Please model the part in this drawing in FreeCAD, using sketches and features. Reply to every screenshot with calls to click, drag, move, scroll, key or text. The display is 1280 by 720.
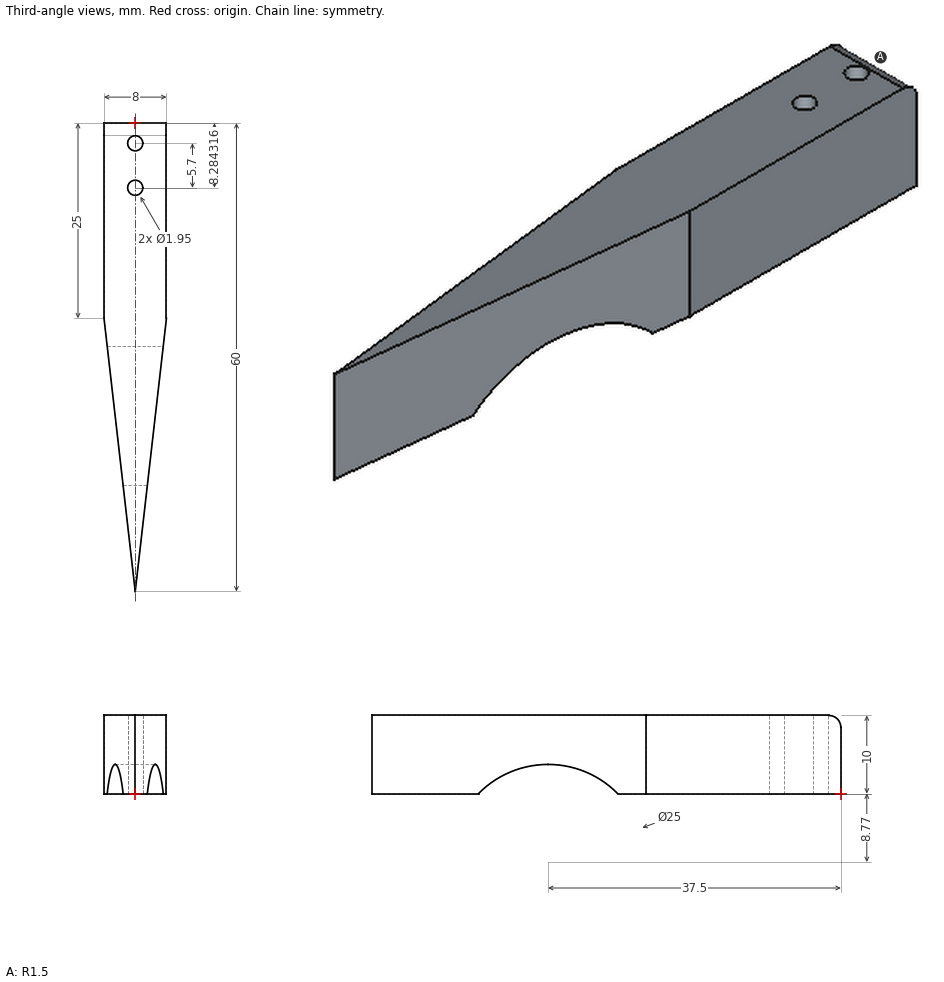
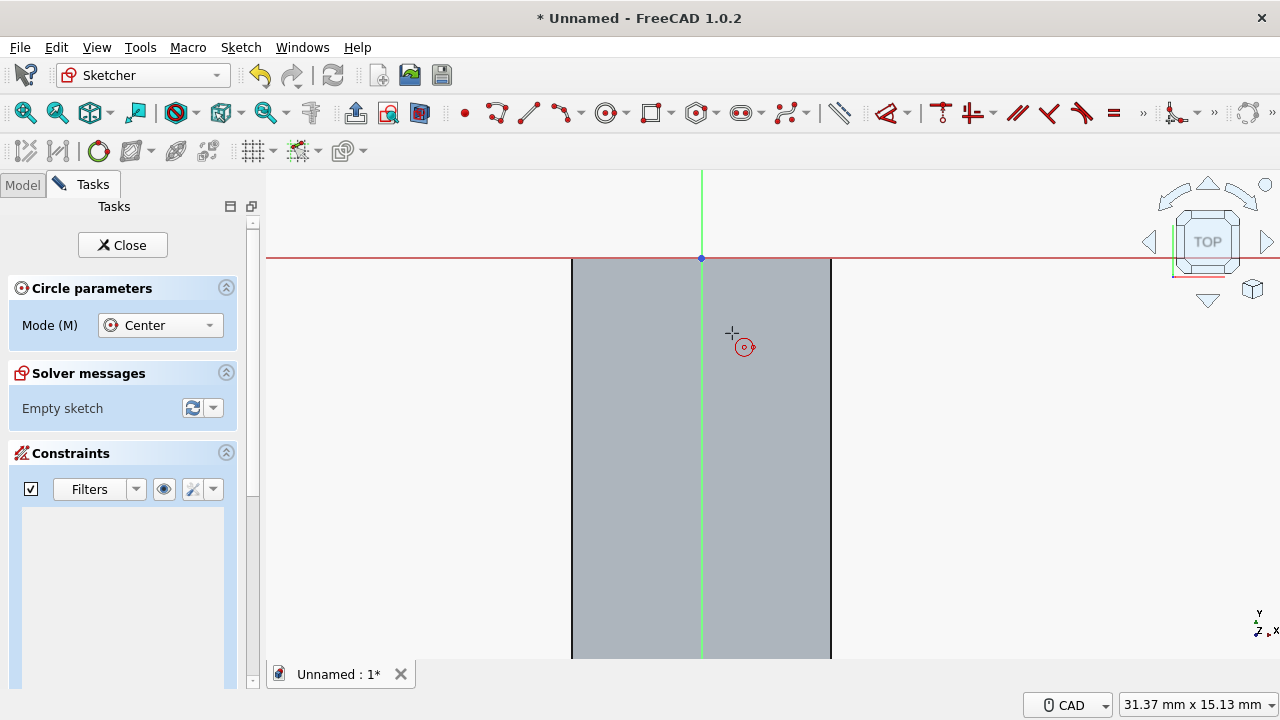
click(702, 526)
move(724, 504)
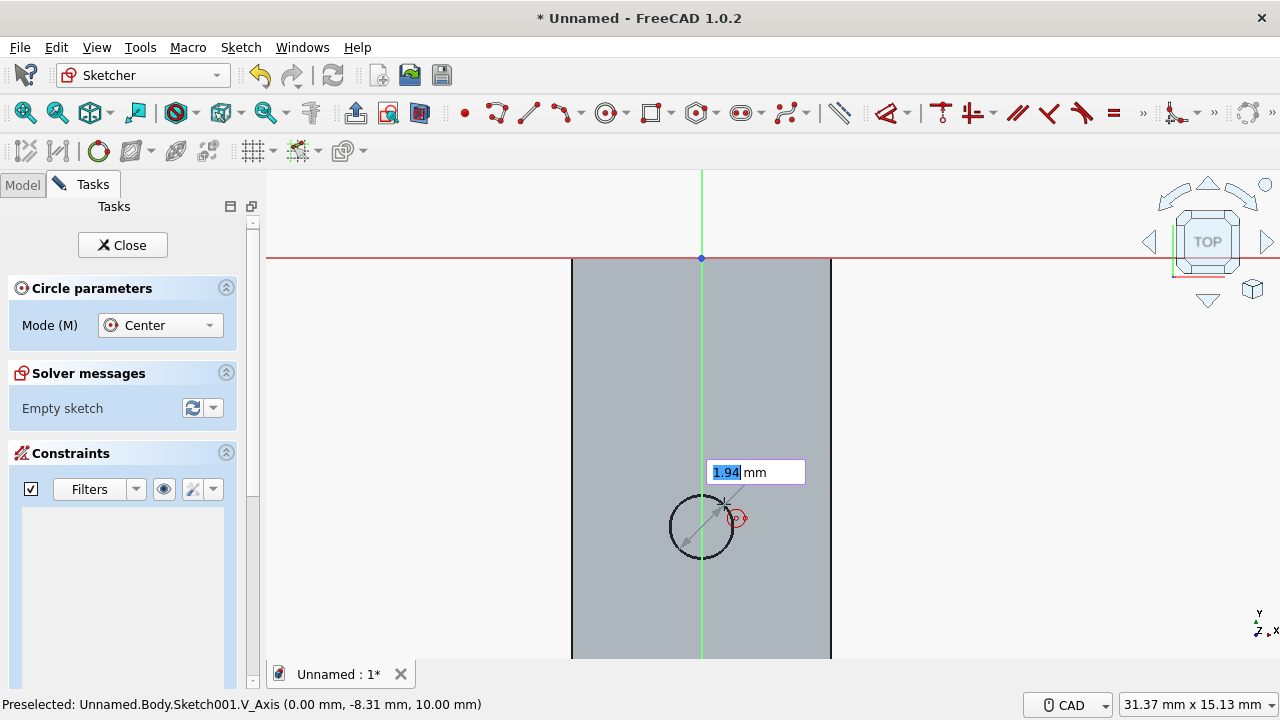
text(1.95)
key(Return)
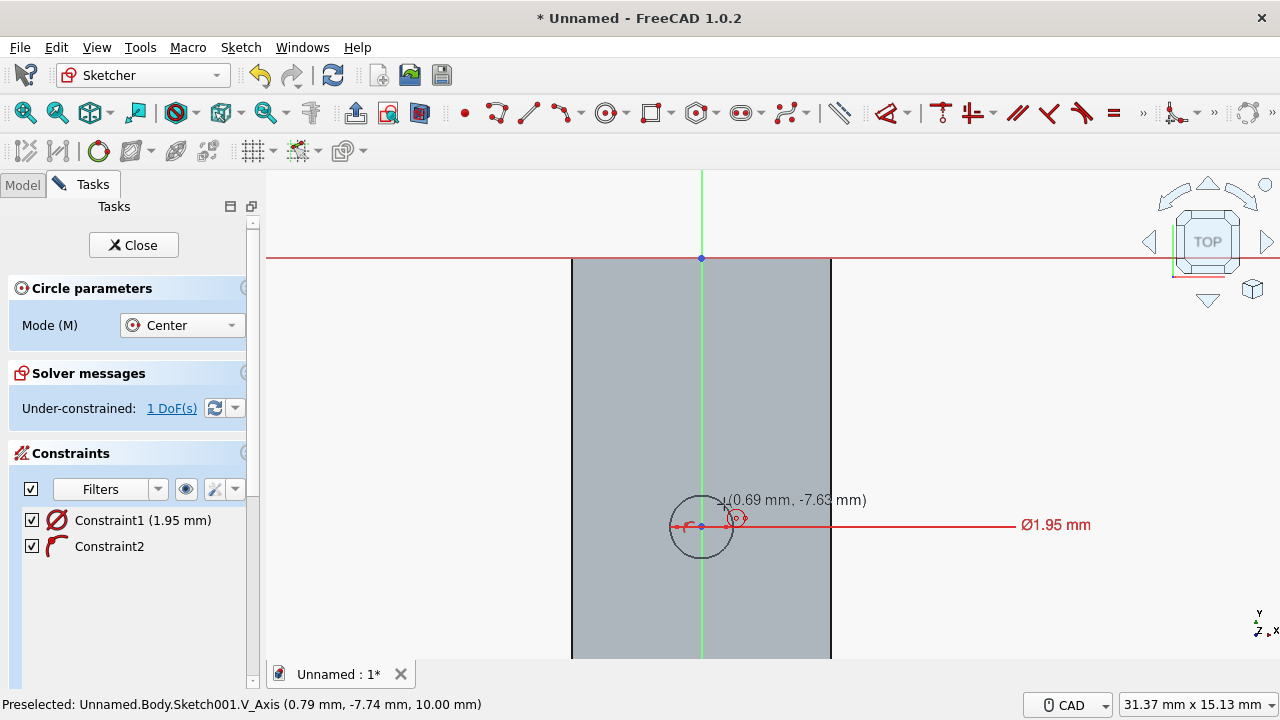
click(702, 342)
move(724, 320)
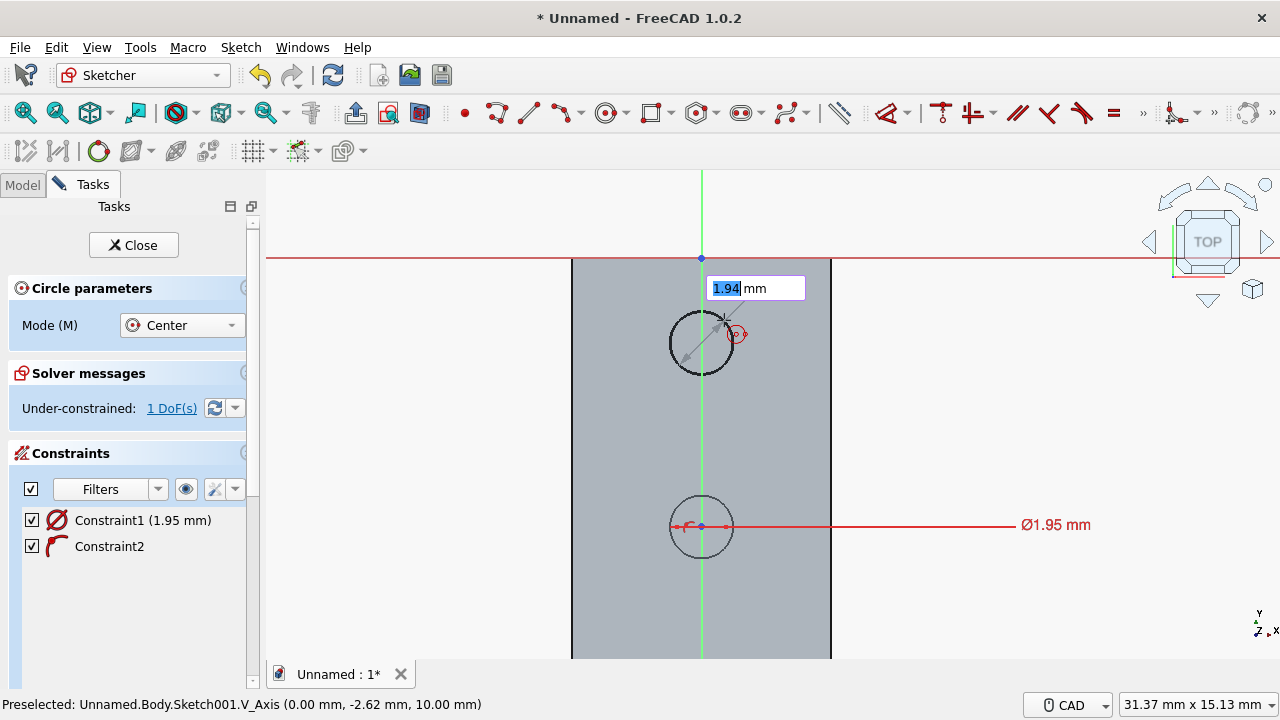
text(1.95)
key(Return)
key(Escape)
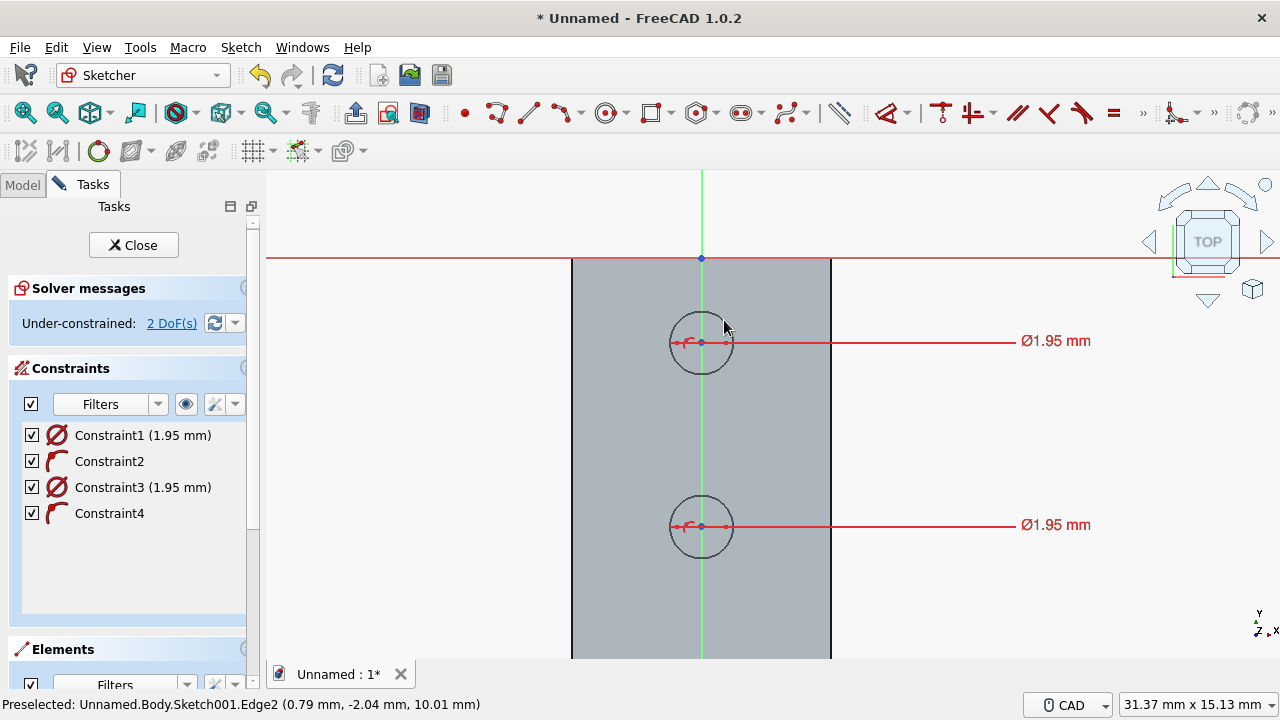
click(886, 114)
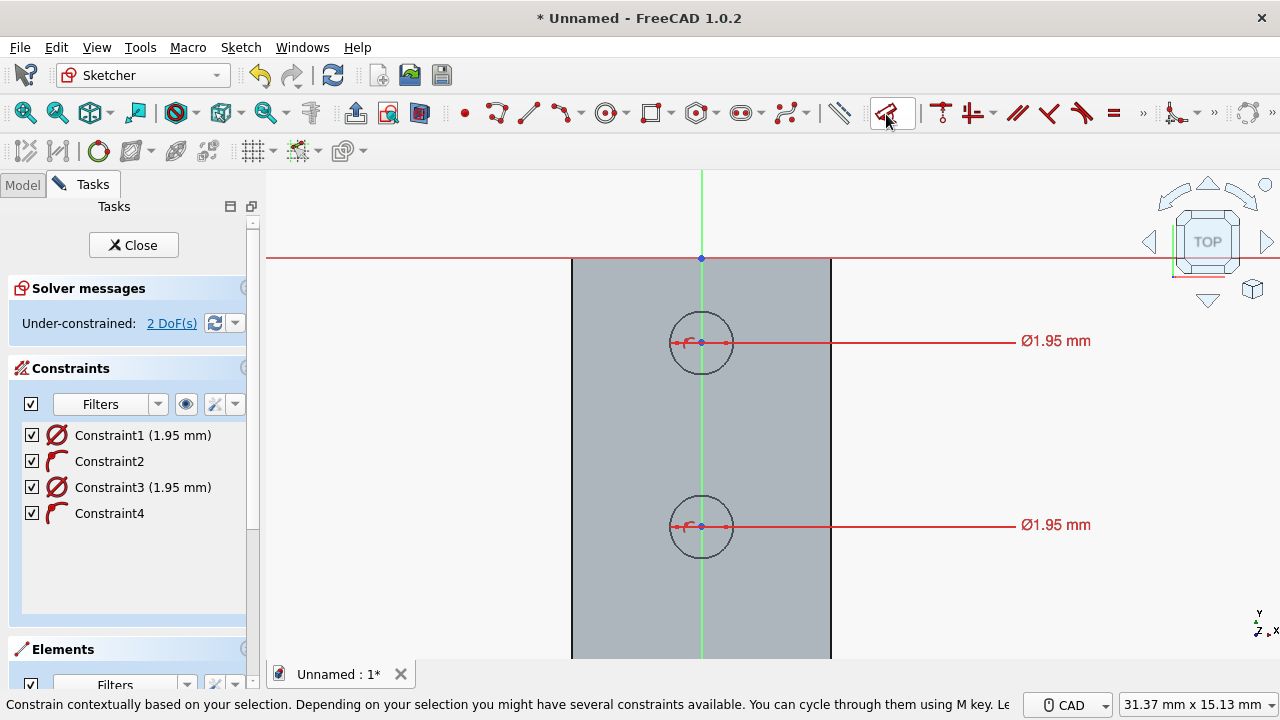
click(702, 527)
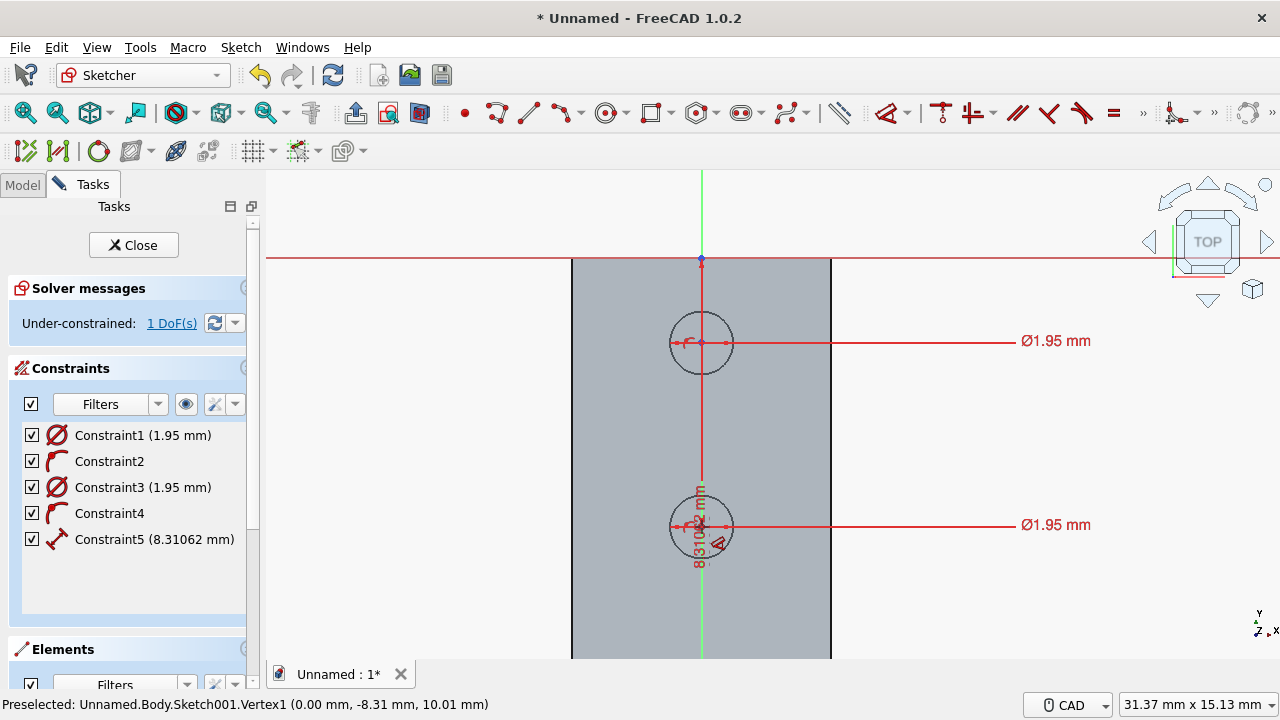
click(702, 343)
click(736, 435)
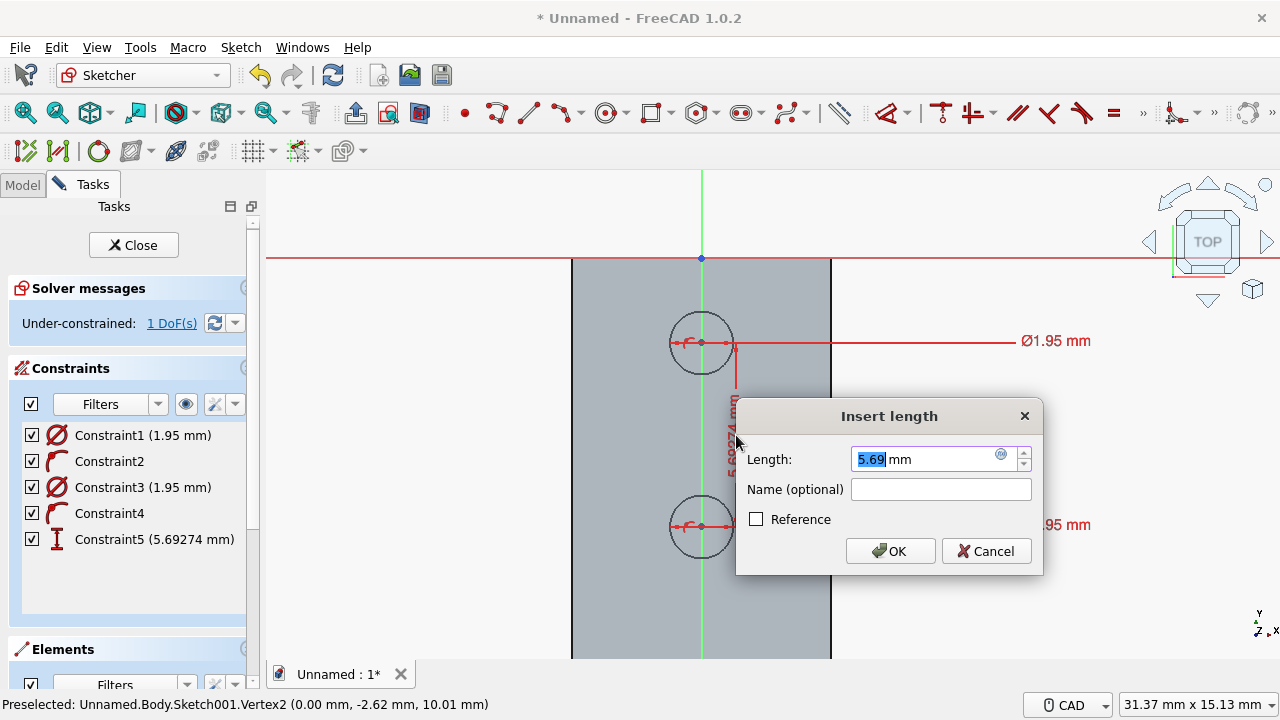
text(5.7)
key(Return)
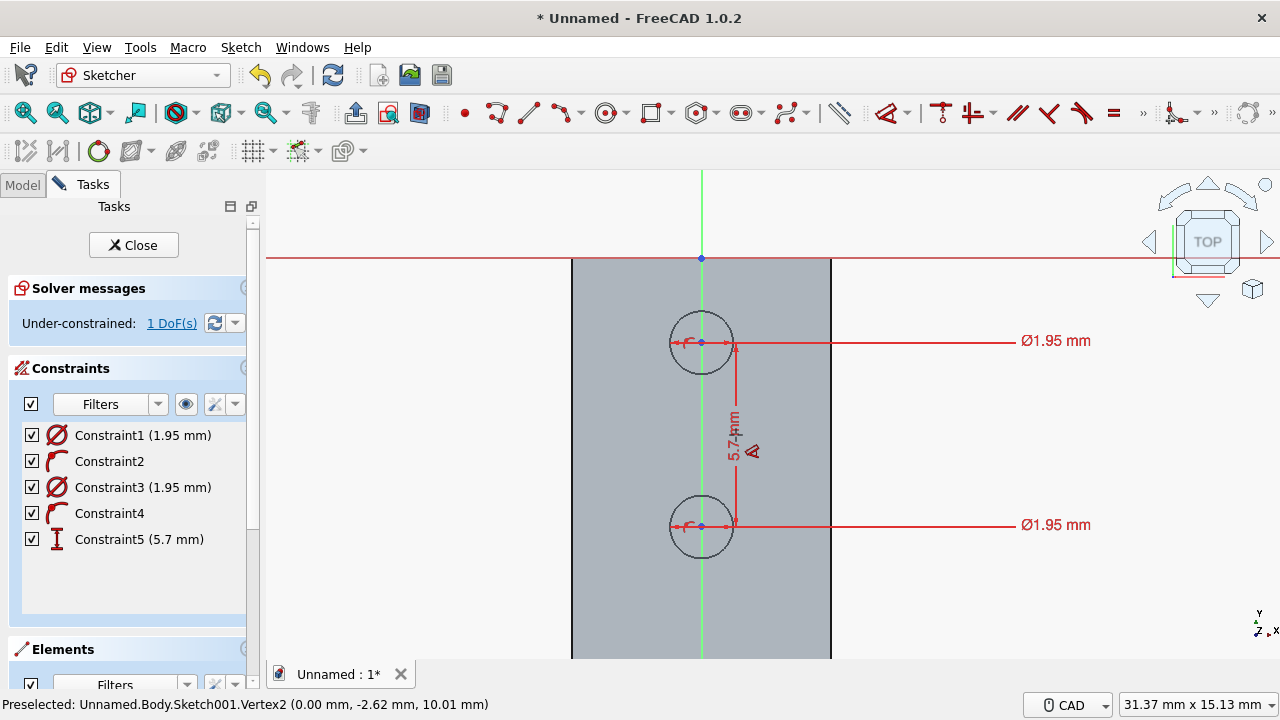
click(702, 527)
click(736, 393)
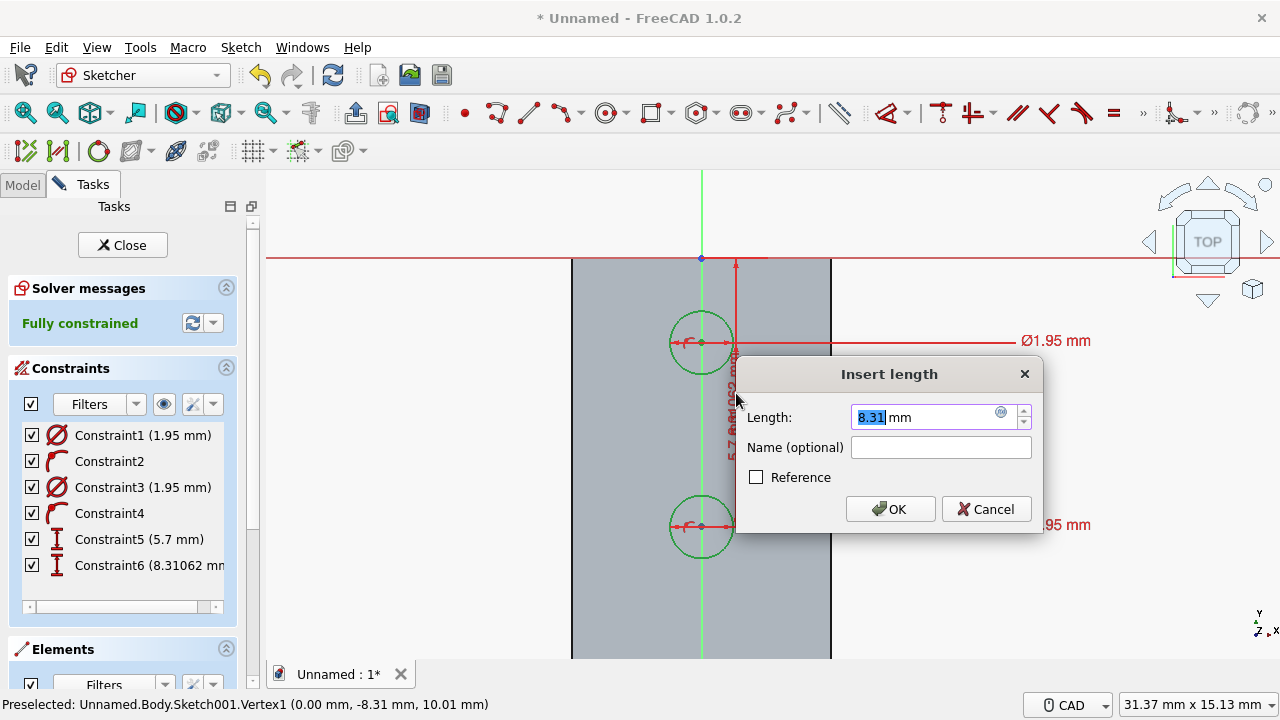
text(8.284316)
key(Return)
key(Escape)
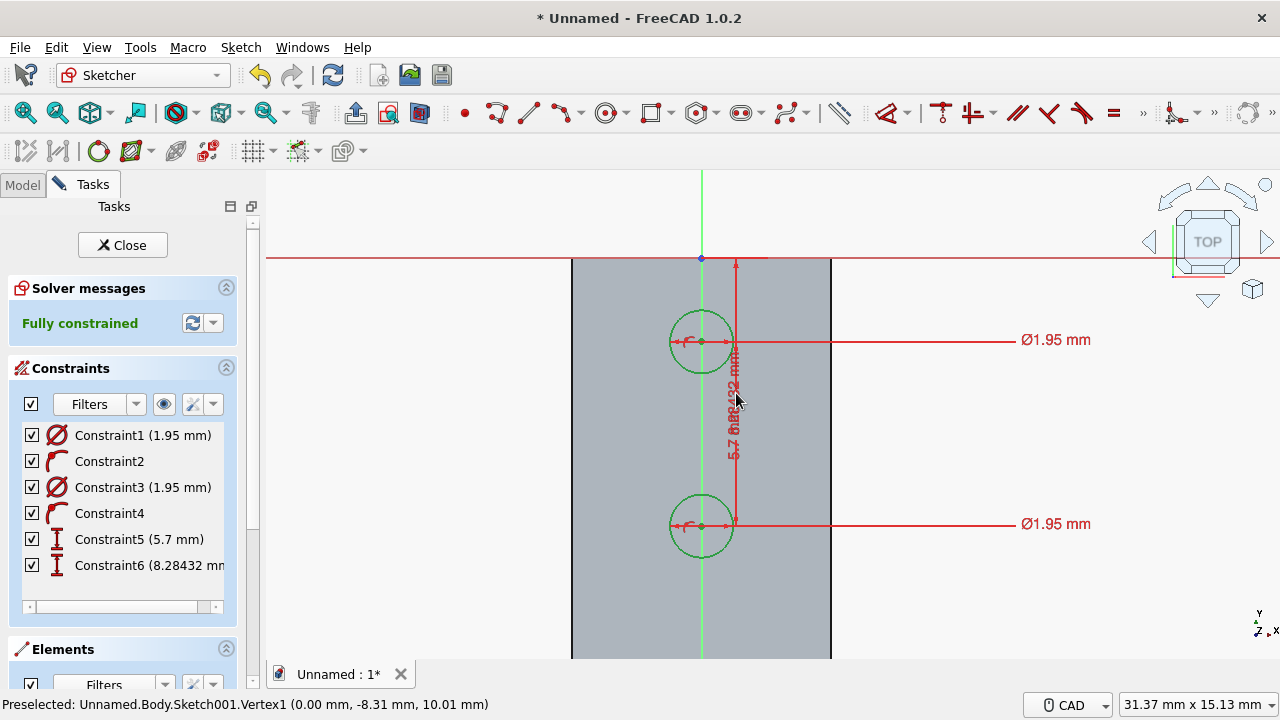
click(123, 245)